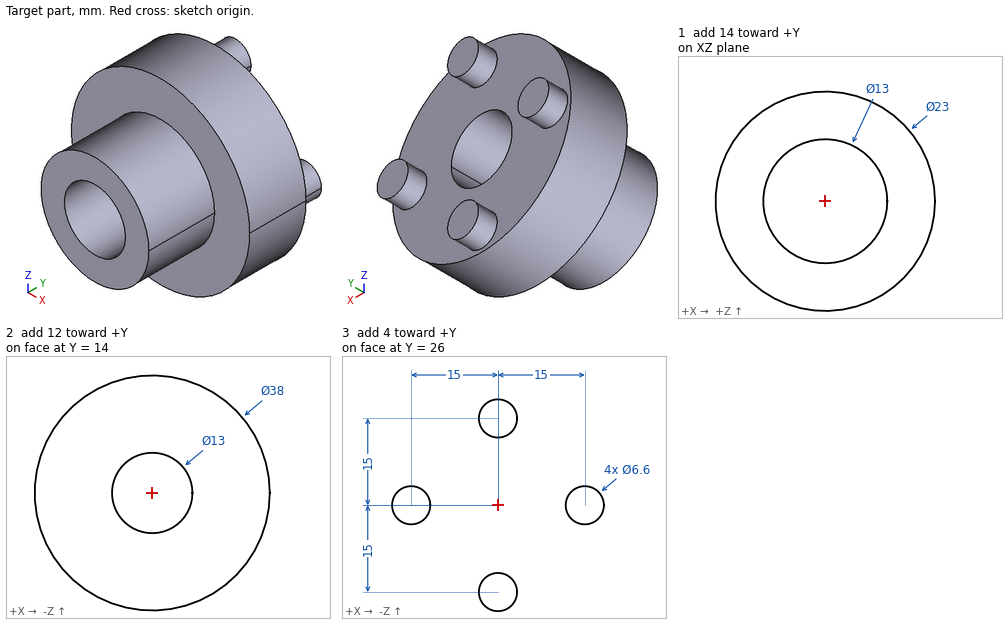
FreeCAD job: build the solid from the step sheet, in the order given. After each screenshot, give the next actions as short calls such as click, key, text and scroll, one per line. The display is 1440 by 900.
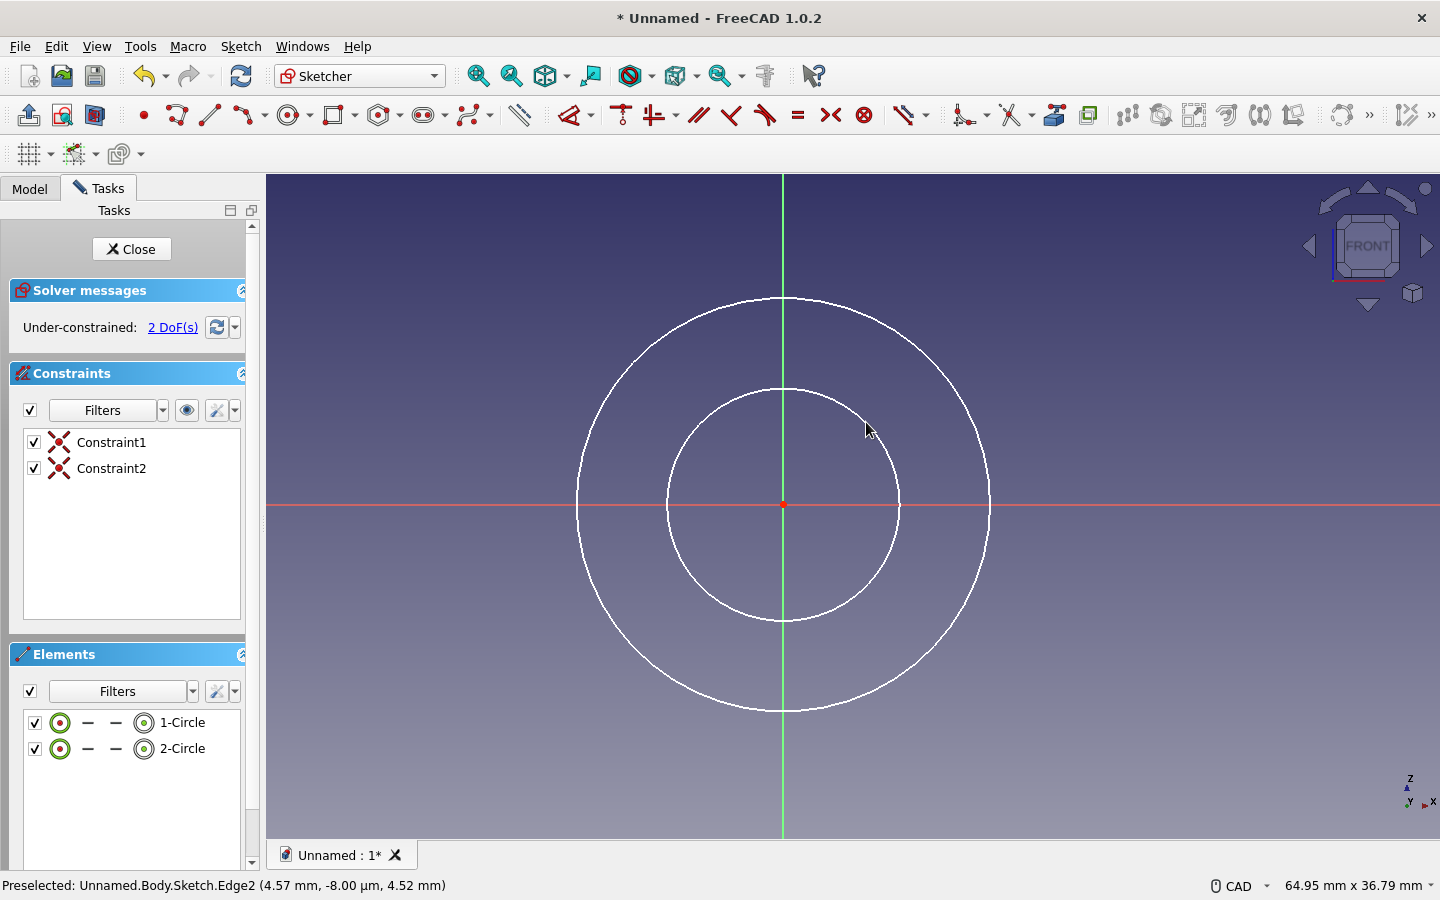
key(d)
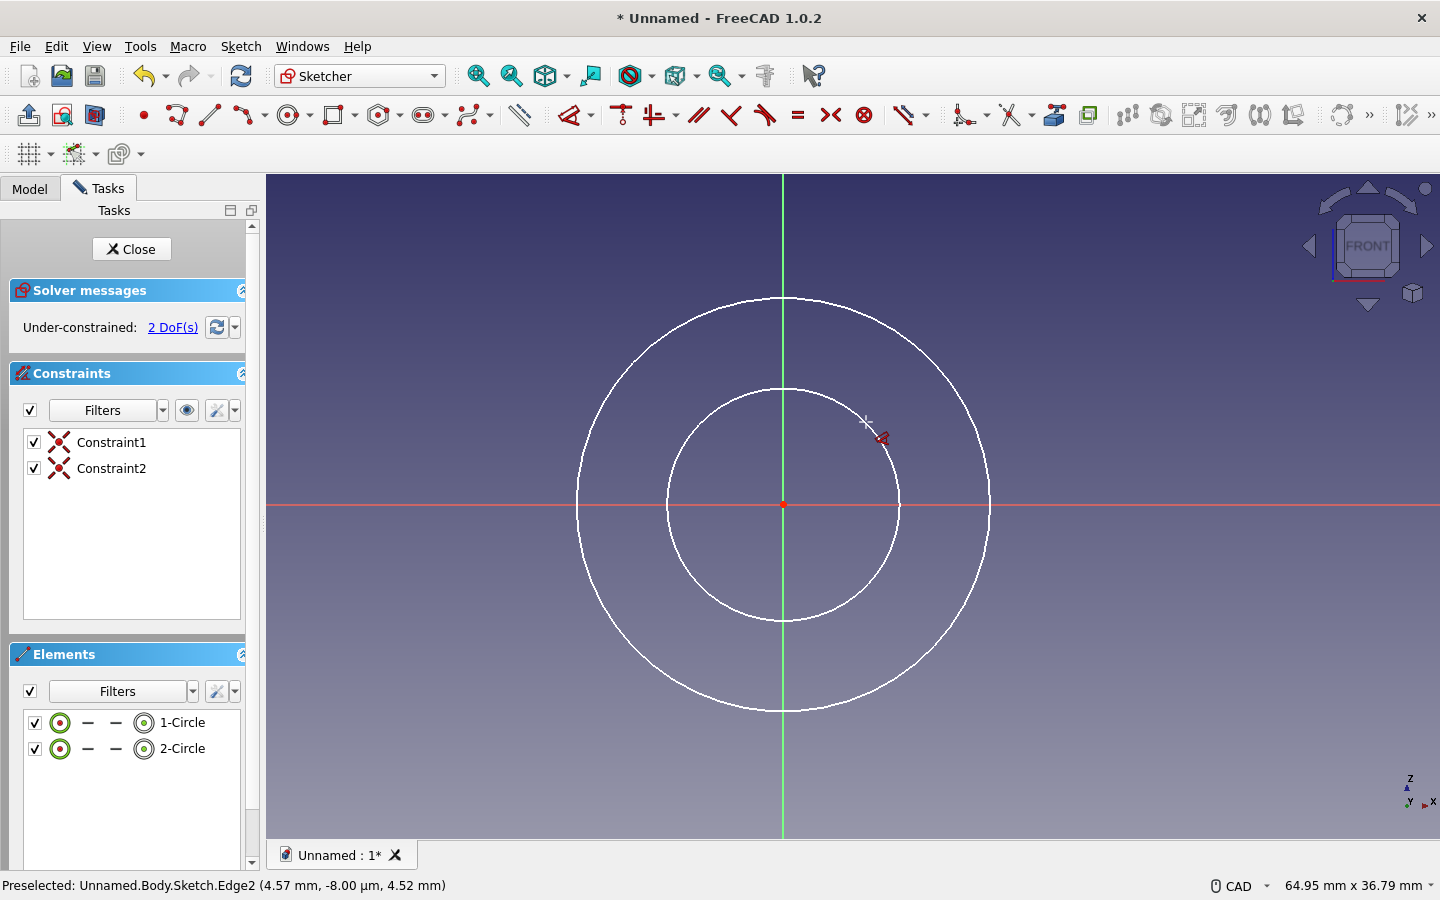
click(929, 358)
click(952, 335)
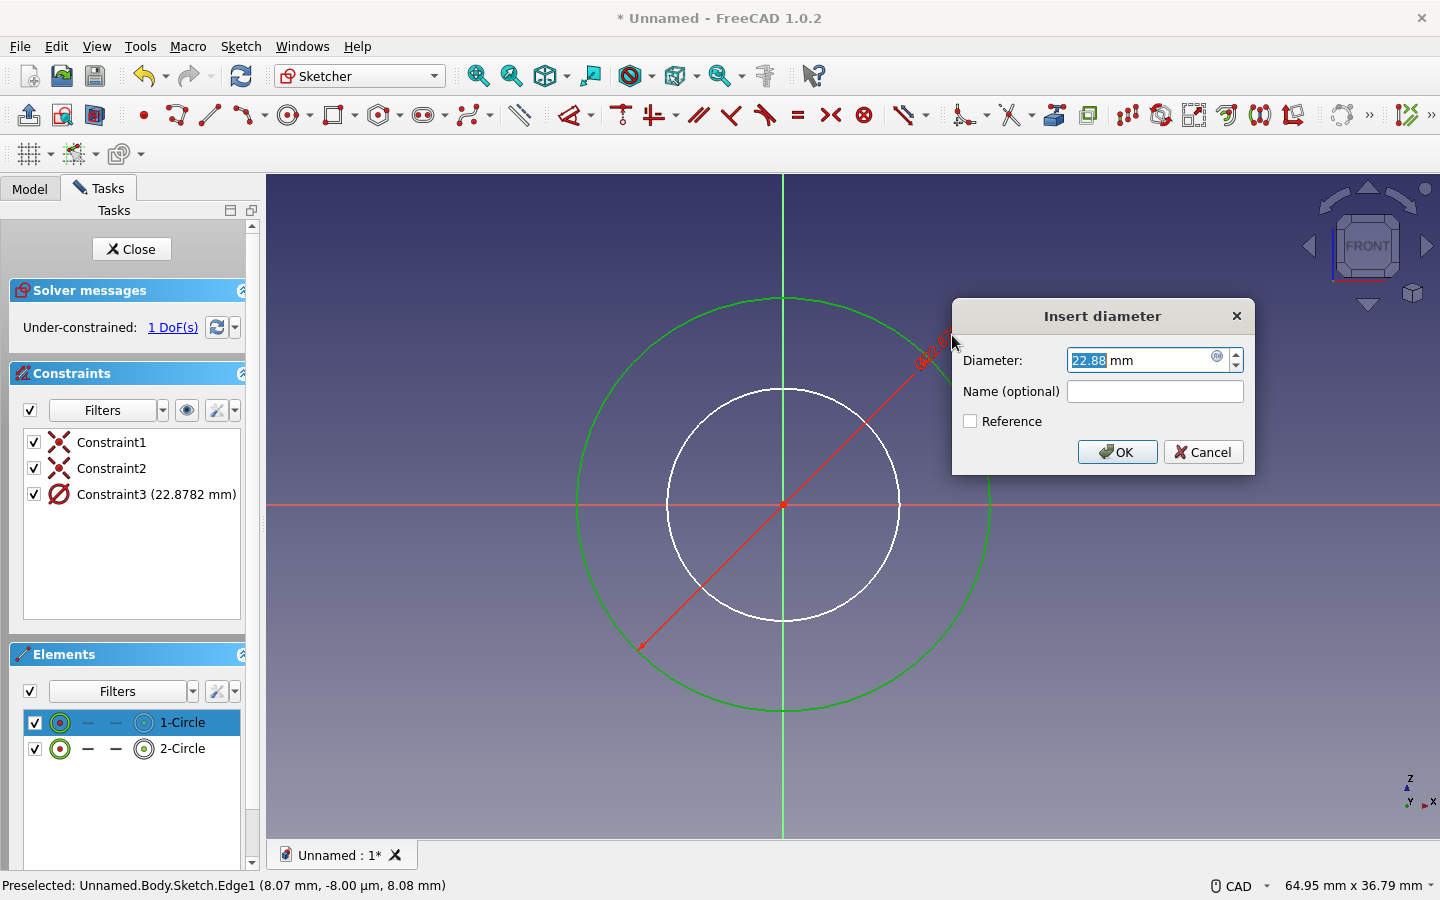
text(23)
key(Return)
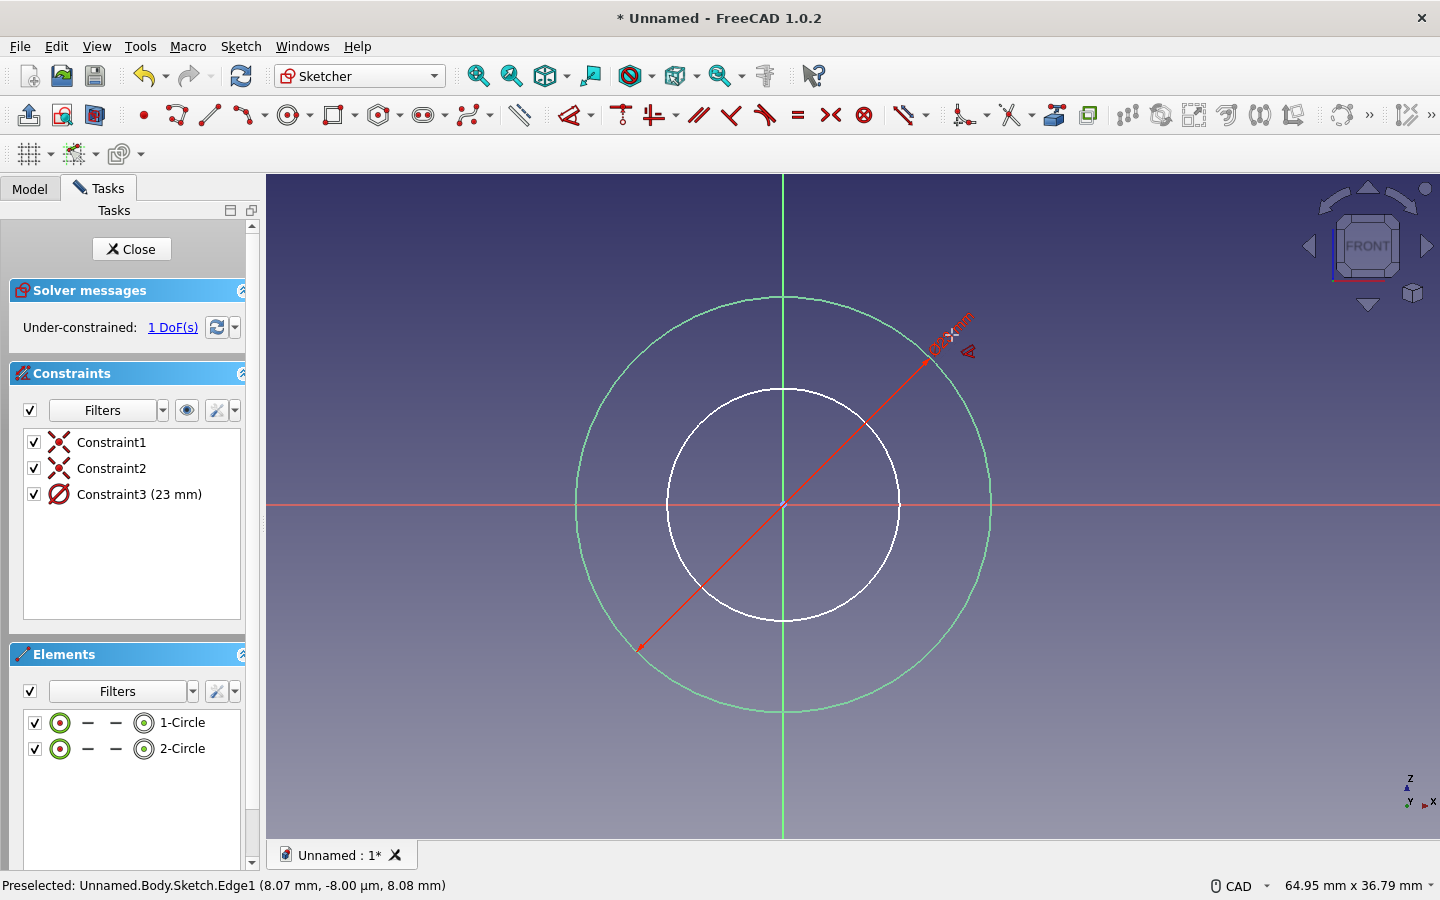
click(865, 422)
click(887, 399)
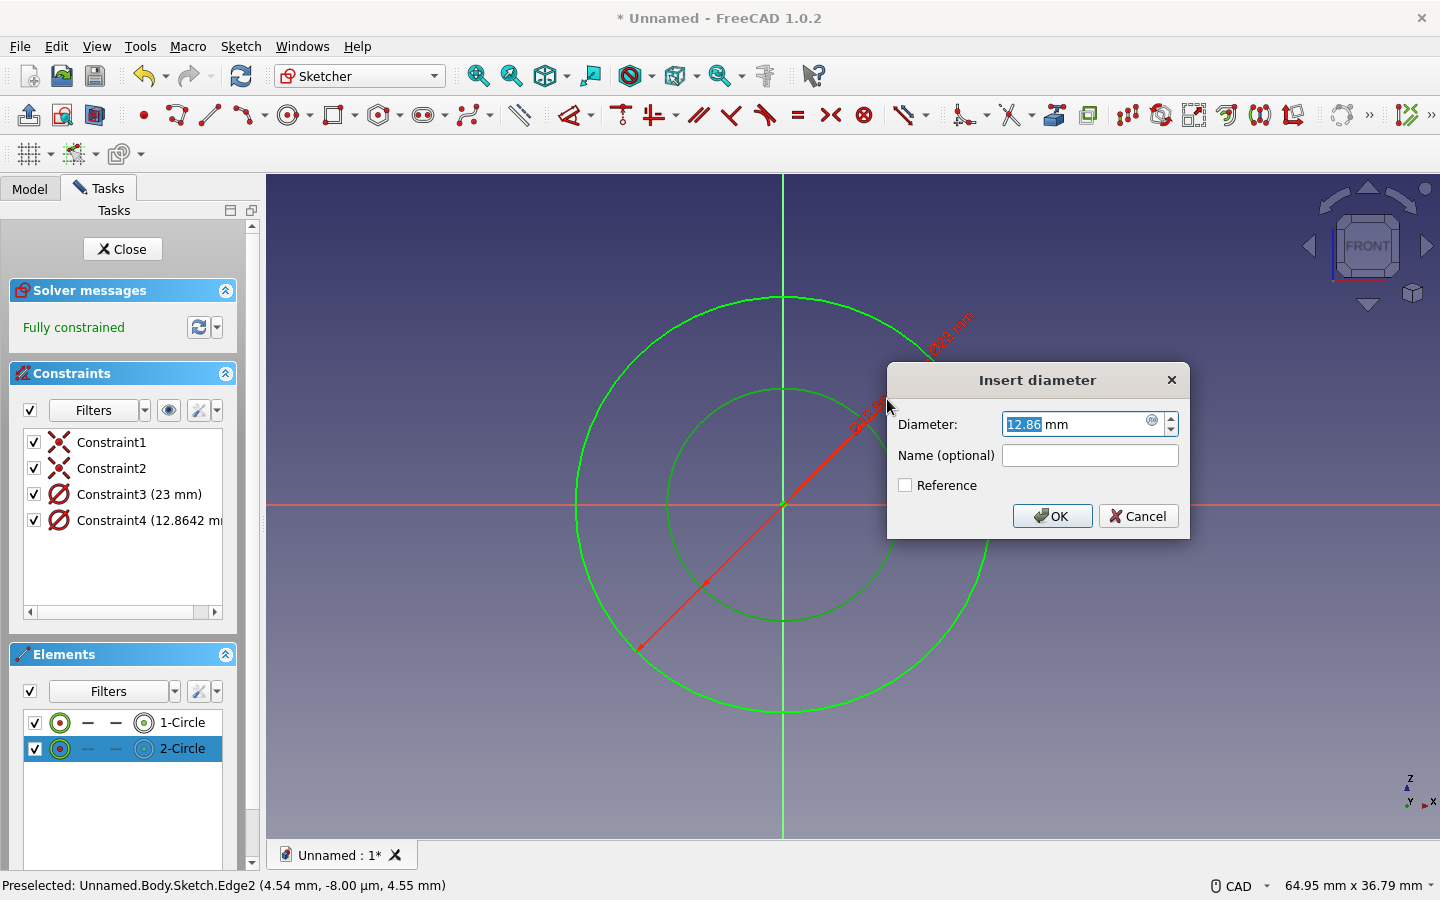
text(13)
key(Return)
key(Escape)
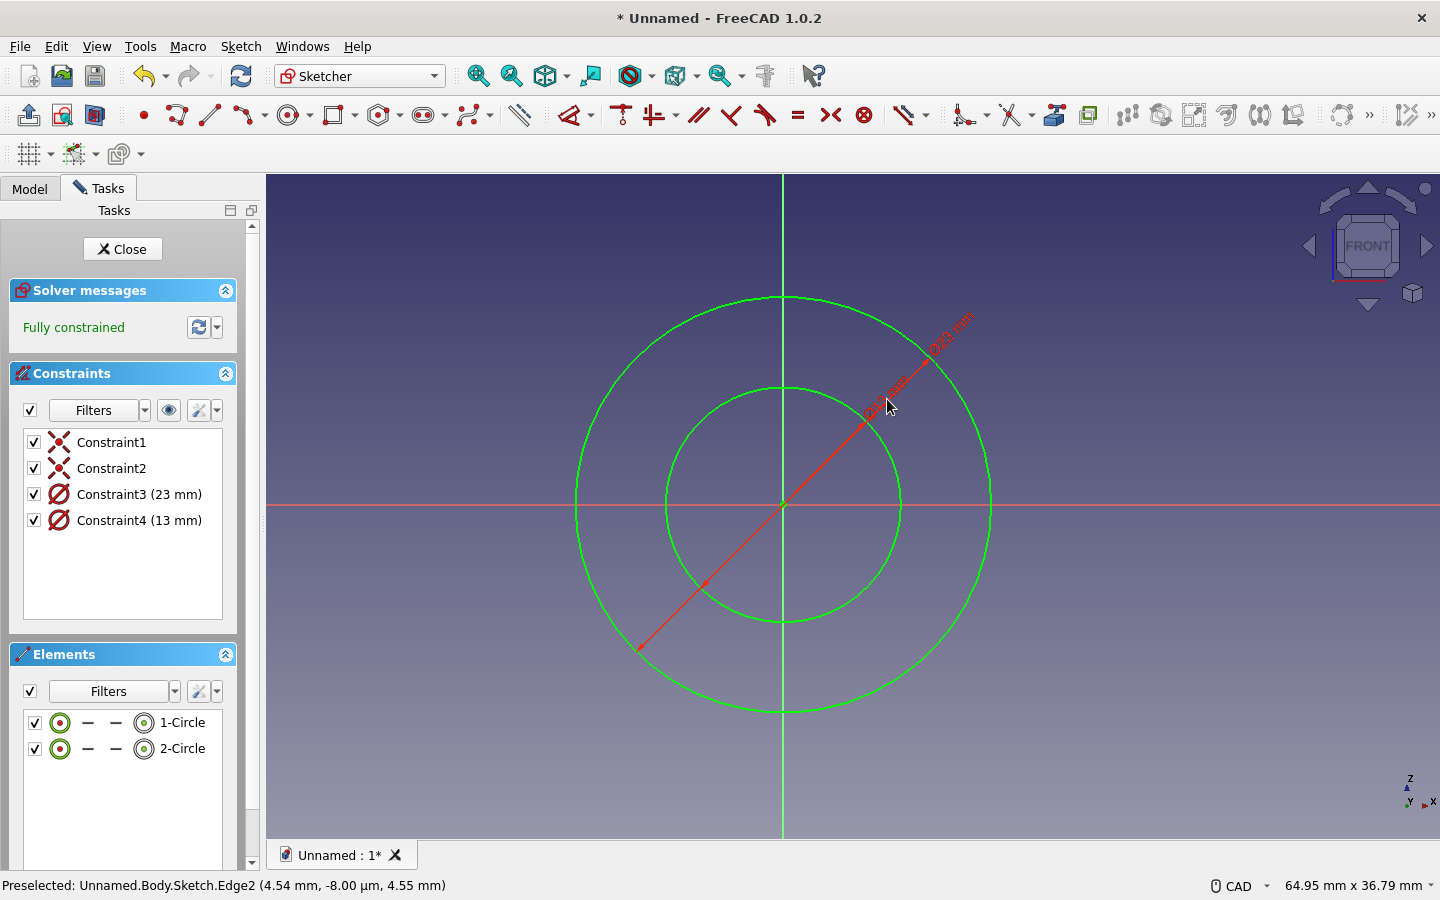
click(123, 249)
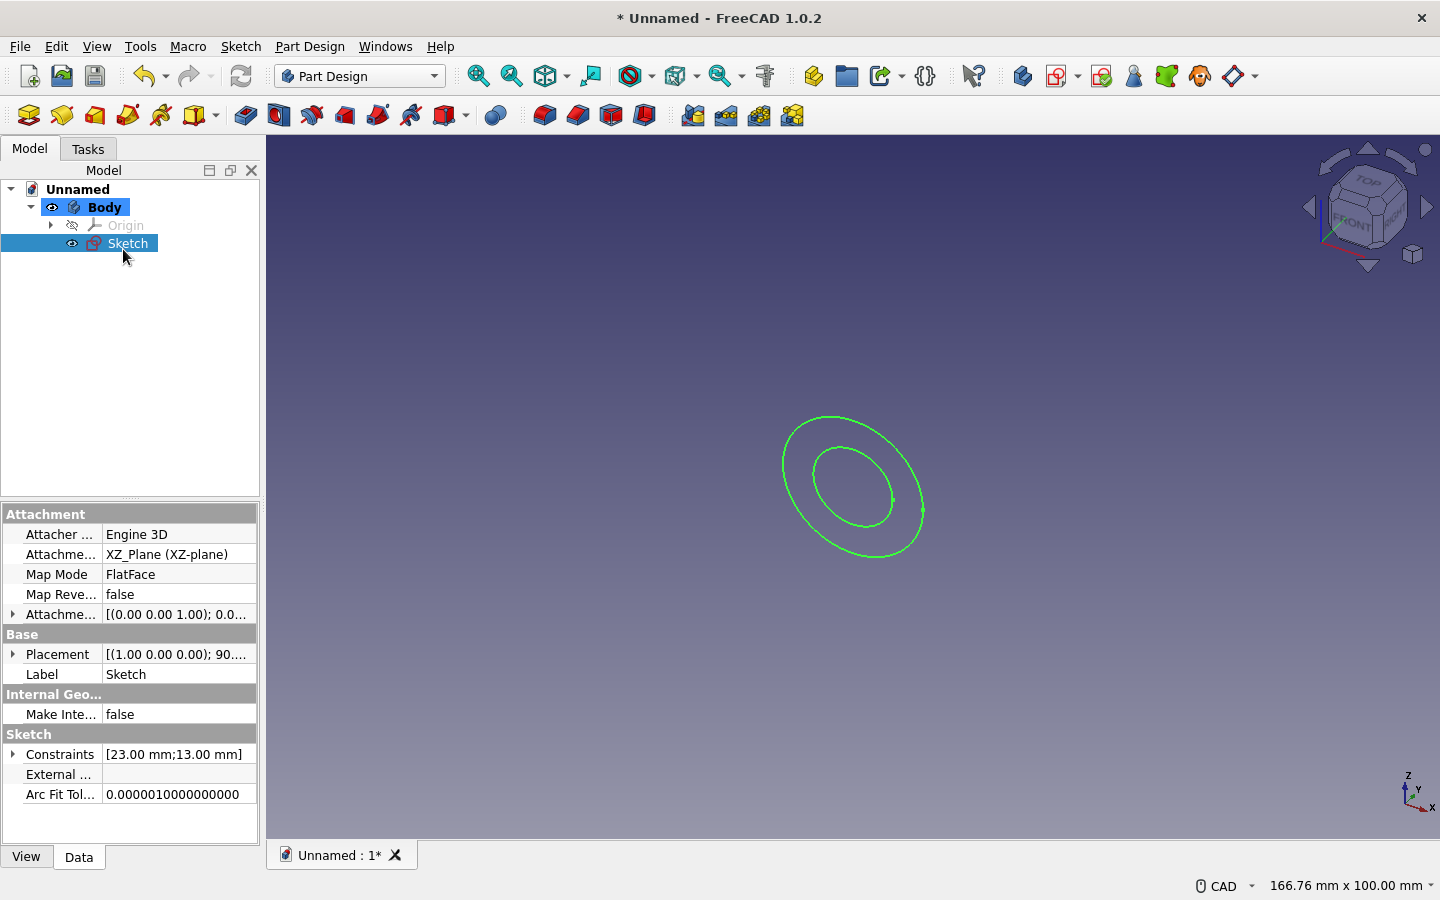
click(29, 116)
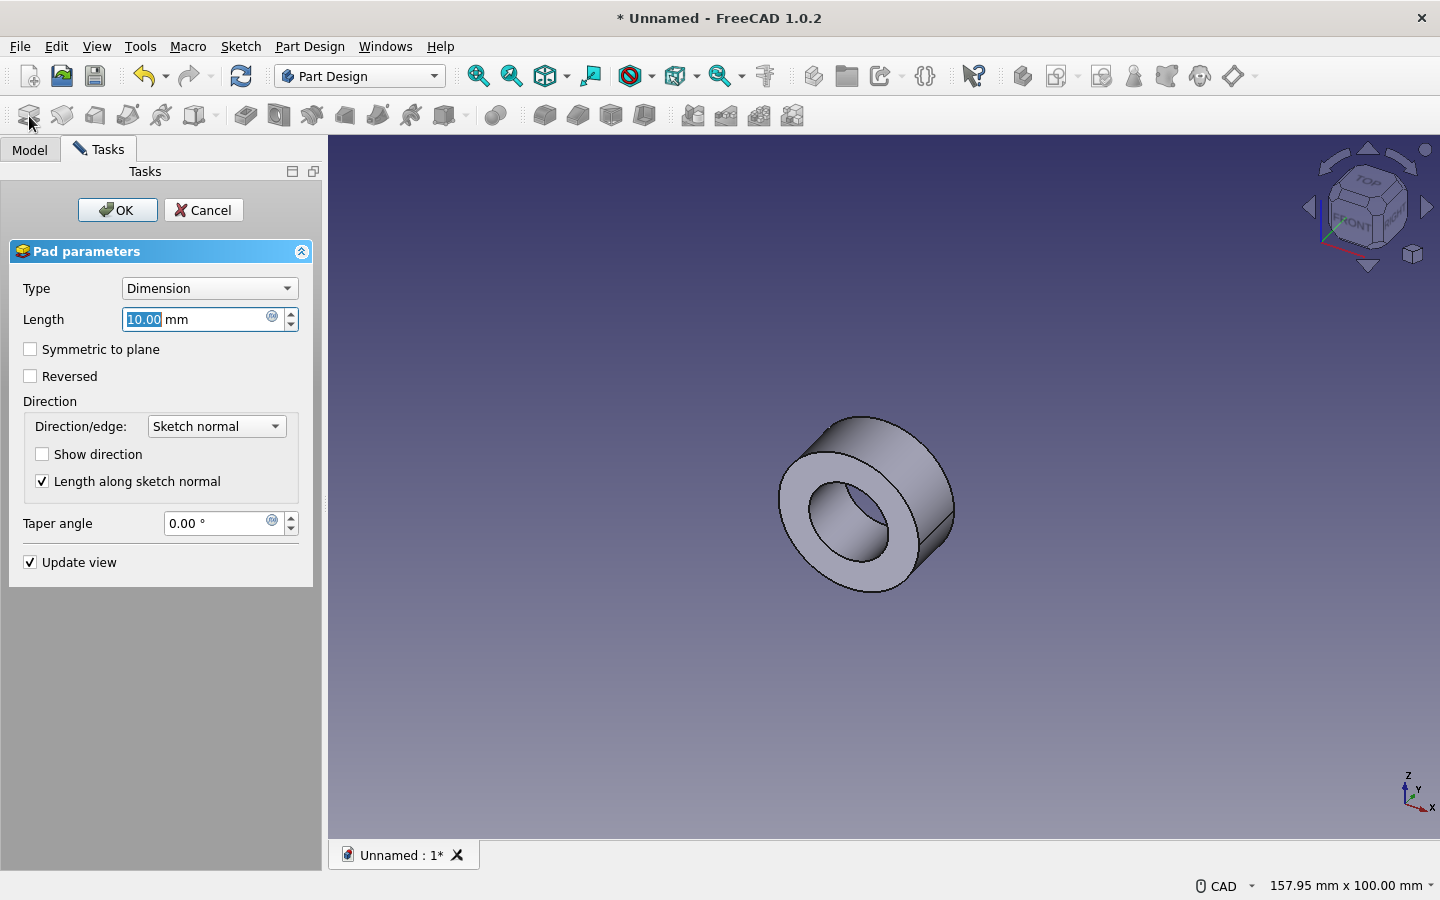
text(14)
key(Tab)